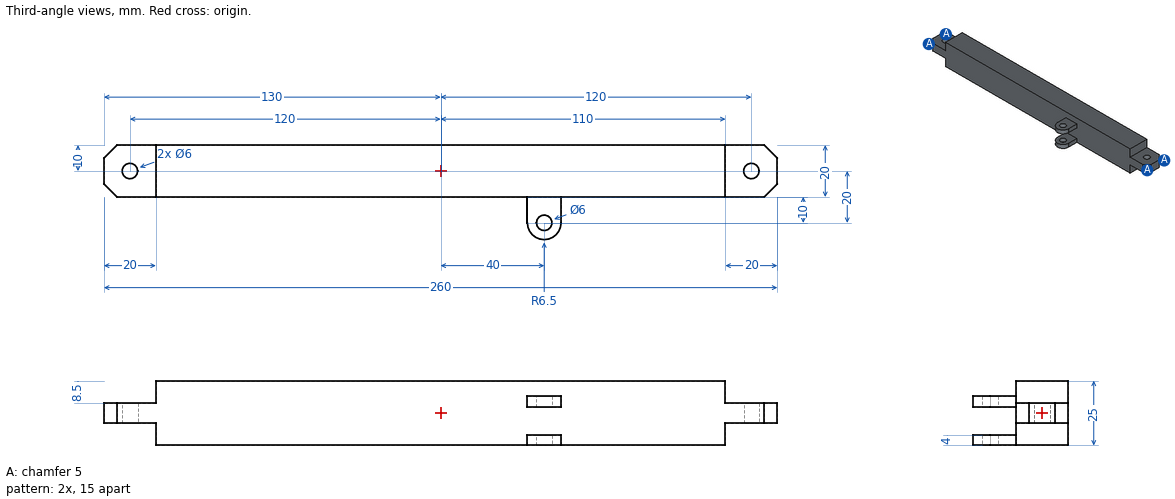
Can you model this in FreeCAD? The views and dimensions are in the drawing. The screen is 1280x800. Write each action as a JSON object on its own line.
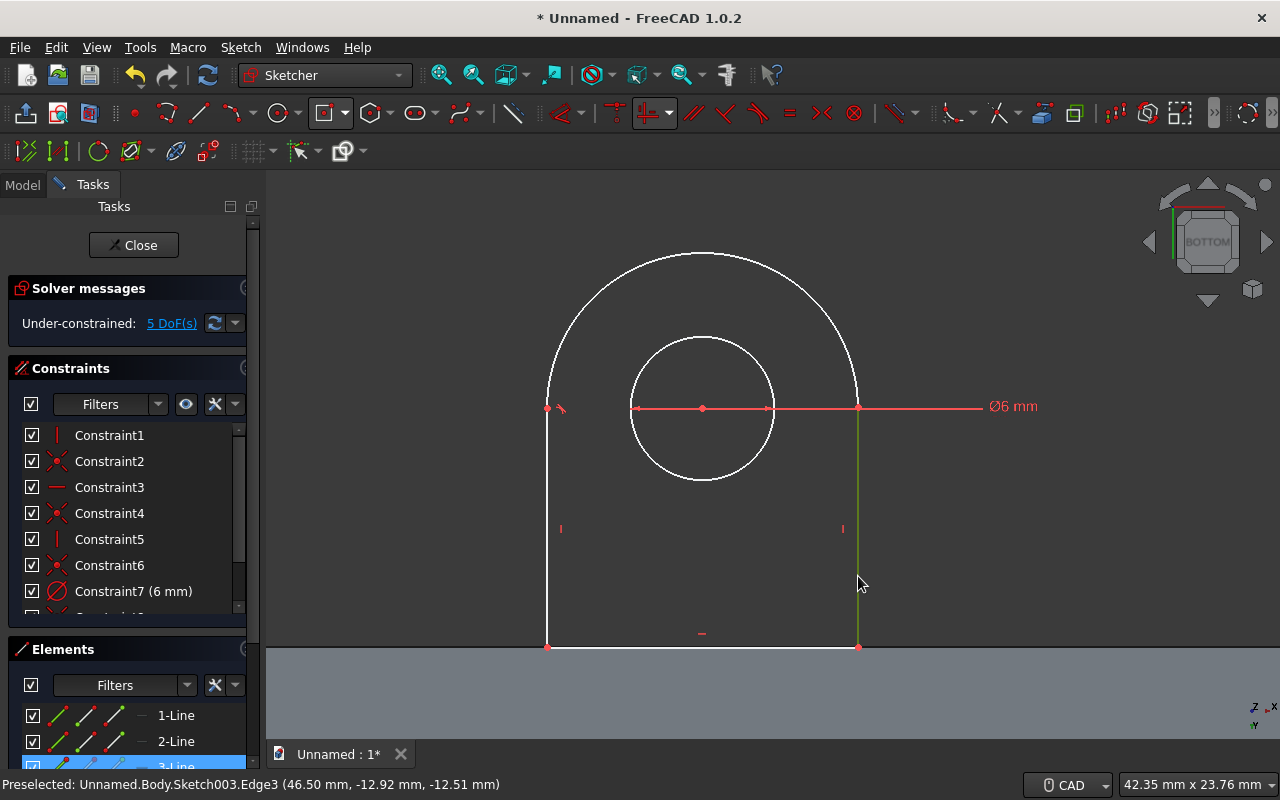
{"action": "left_click", "coordinate": [794, 282]}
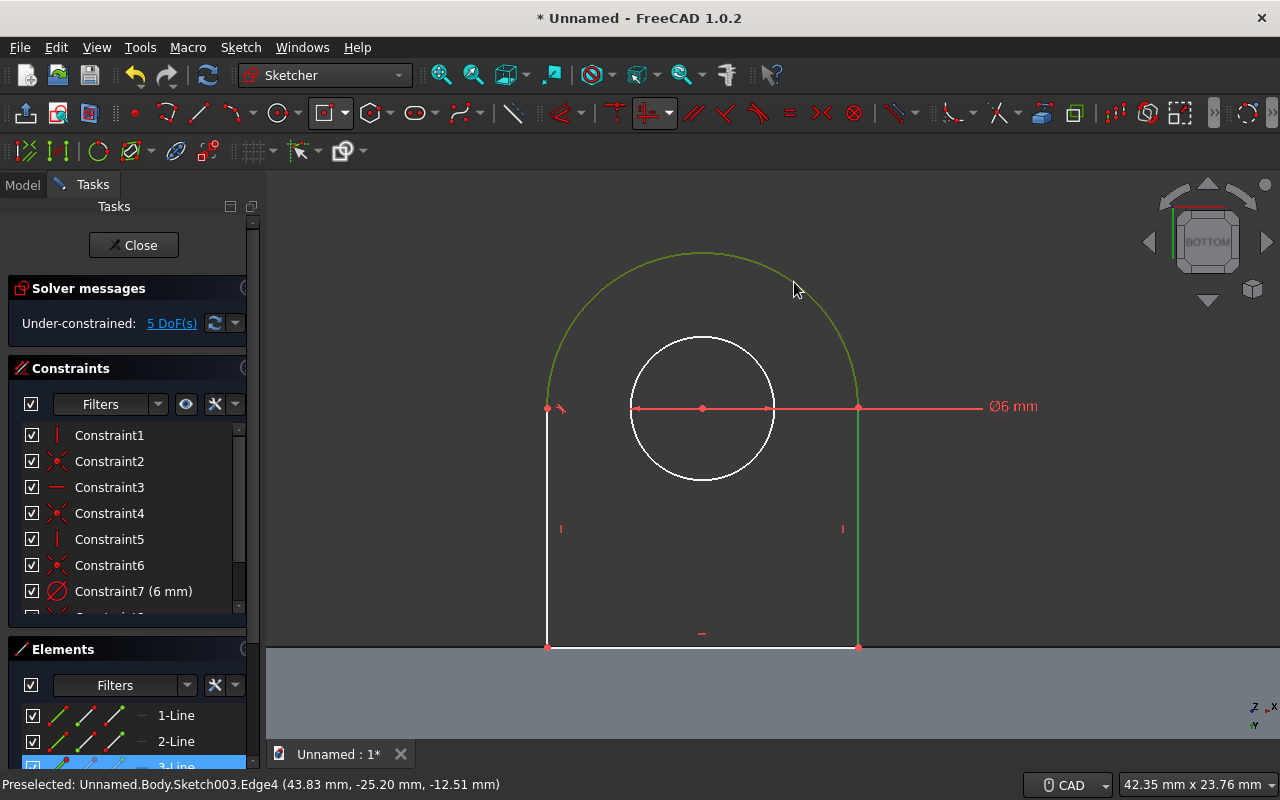
{"action": "left_click", "coordinate": [758, 114]}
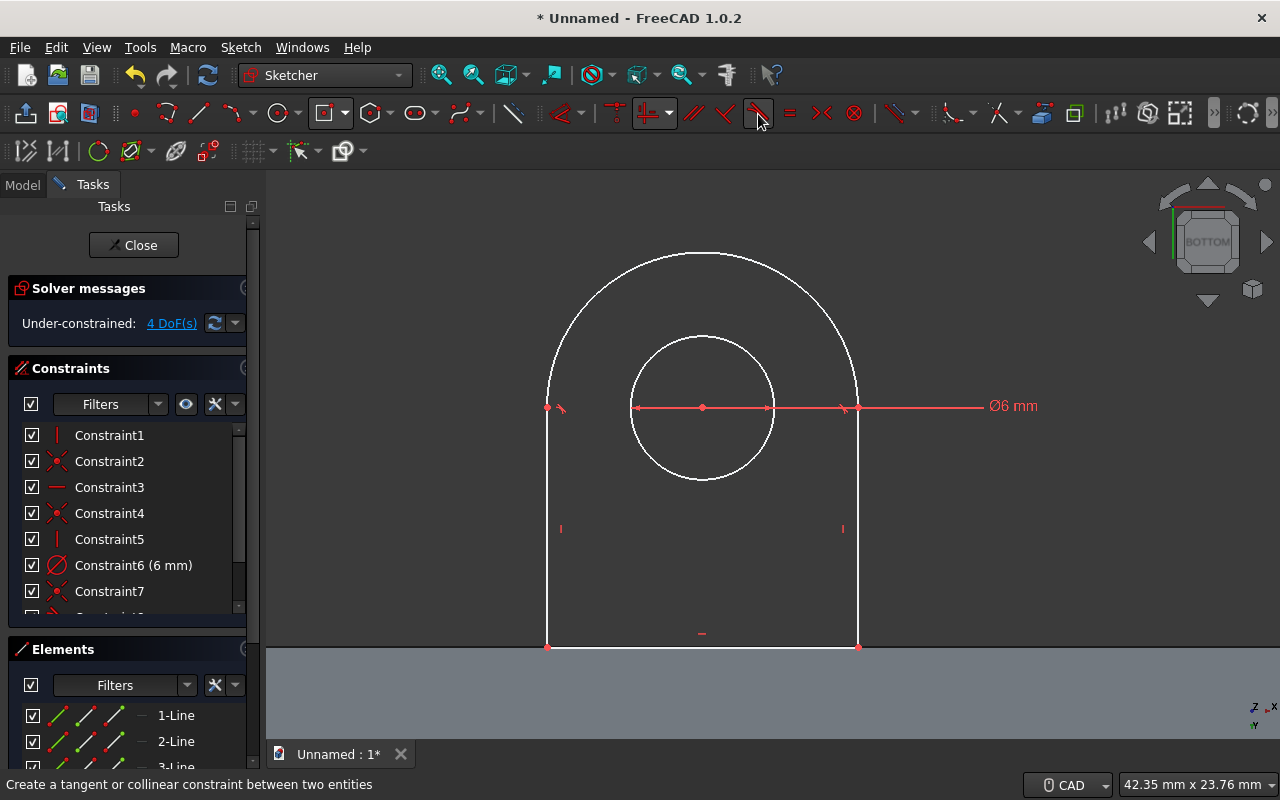
{"action": "left_click", "coordinate": [560, 114]}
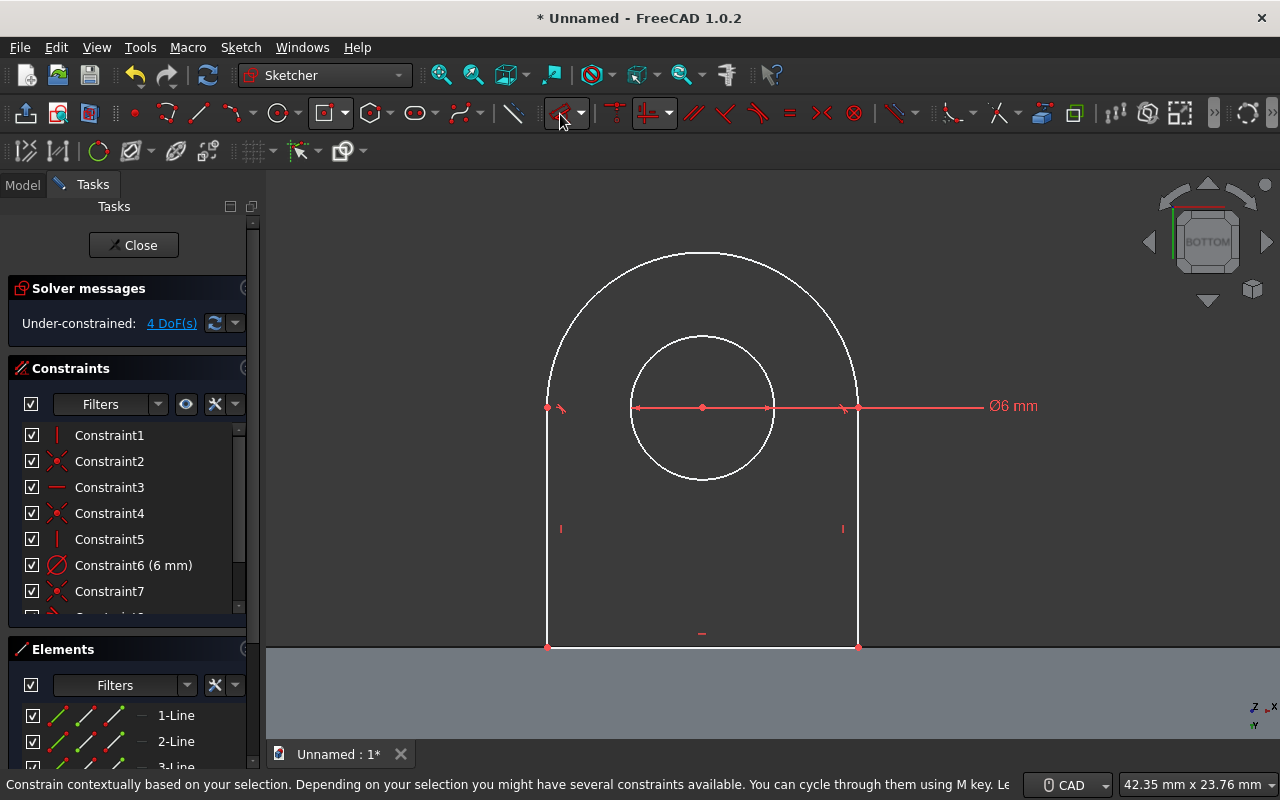
{"action": "left_click", "coordinate": [794, 282]}
{"action": "left_click", "coordinate": [813, 256]}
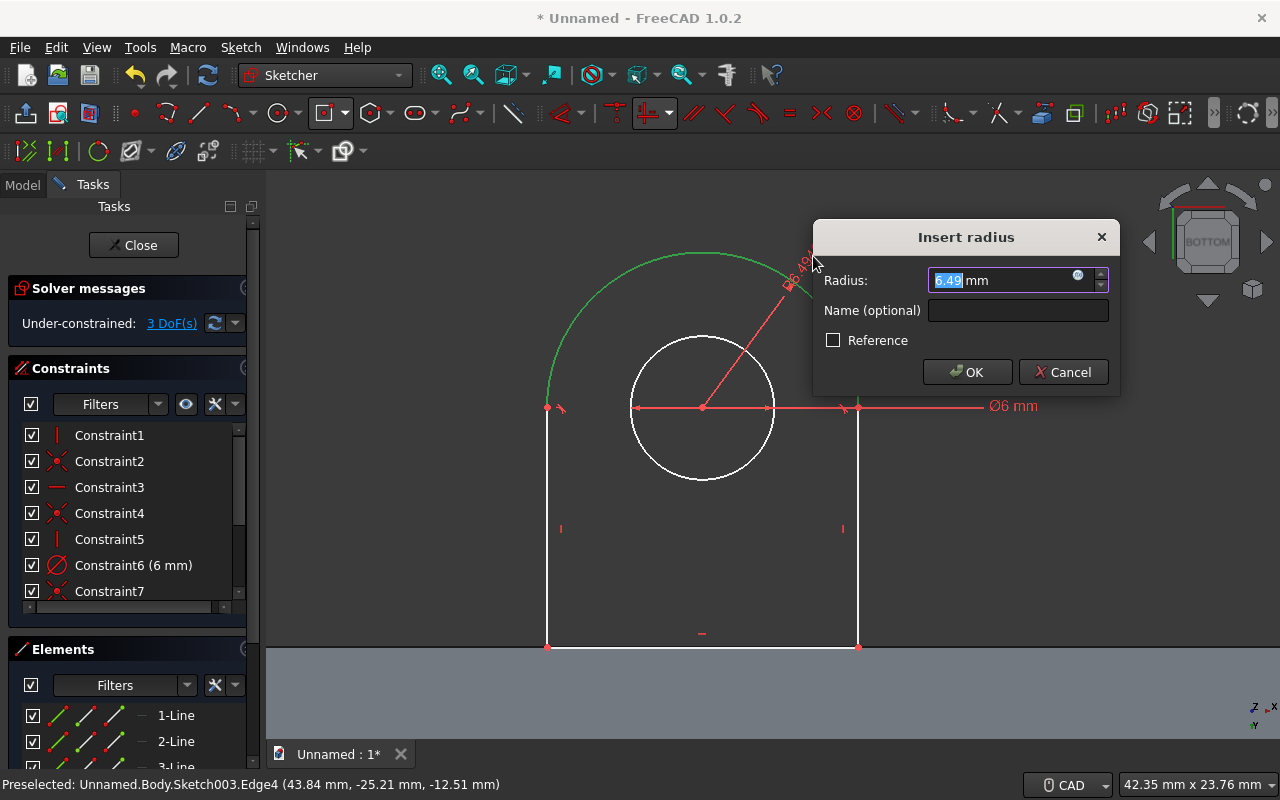
{"action": "type", "text": "6.5"}
{"action": "key", "text": "Return"}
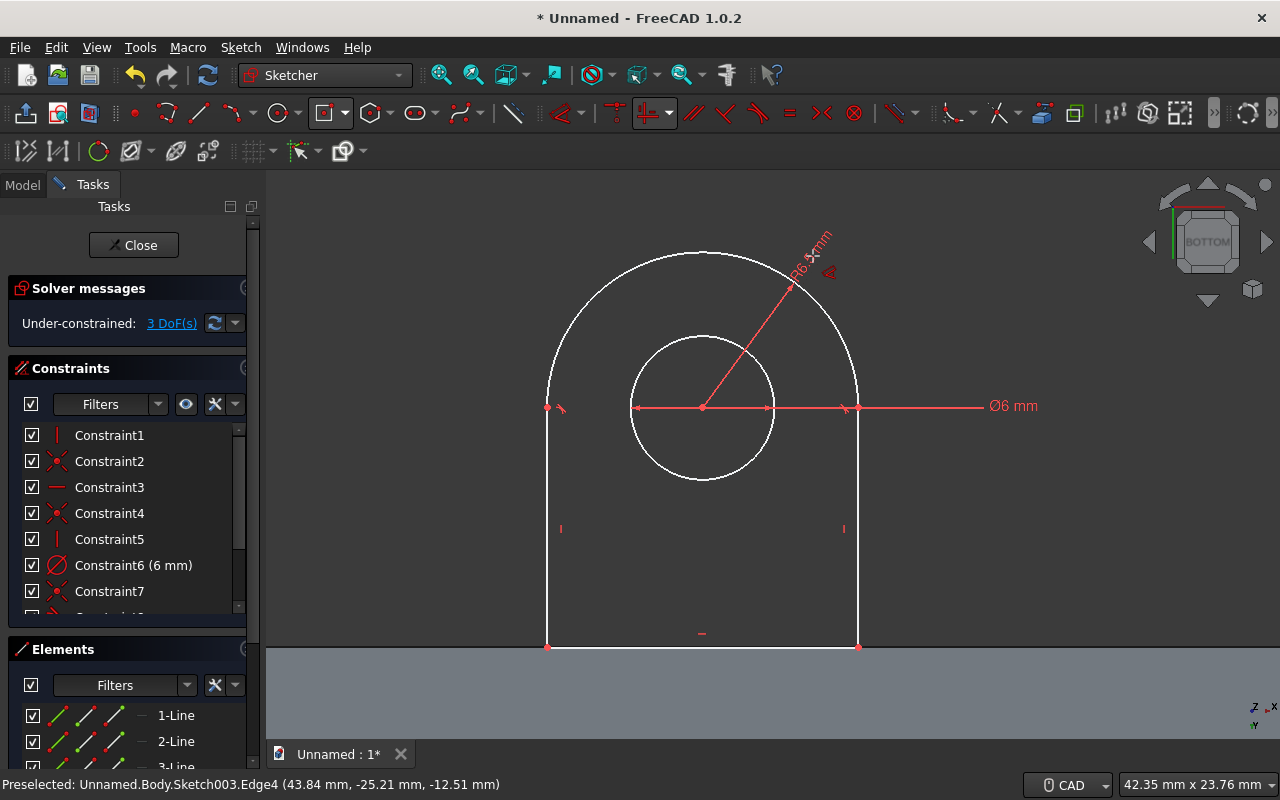
{"action": "left_click", "coordinate": [547, 480]}
{"action": "left_click", "coordinate": [513, 528]}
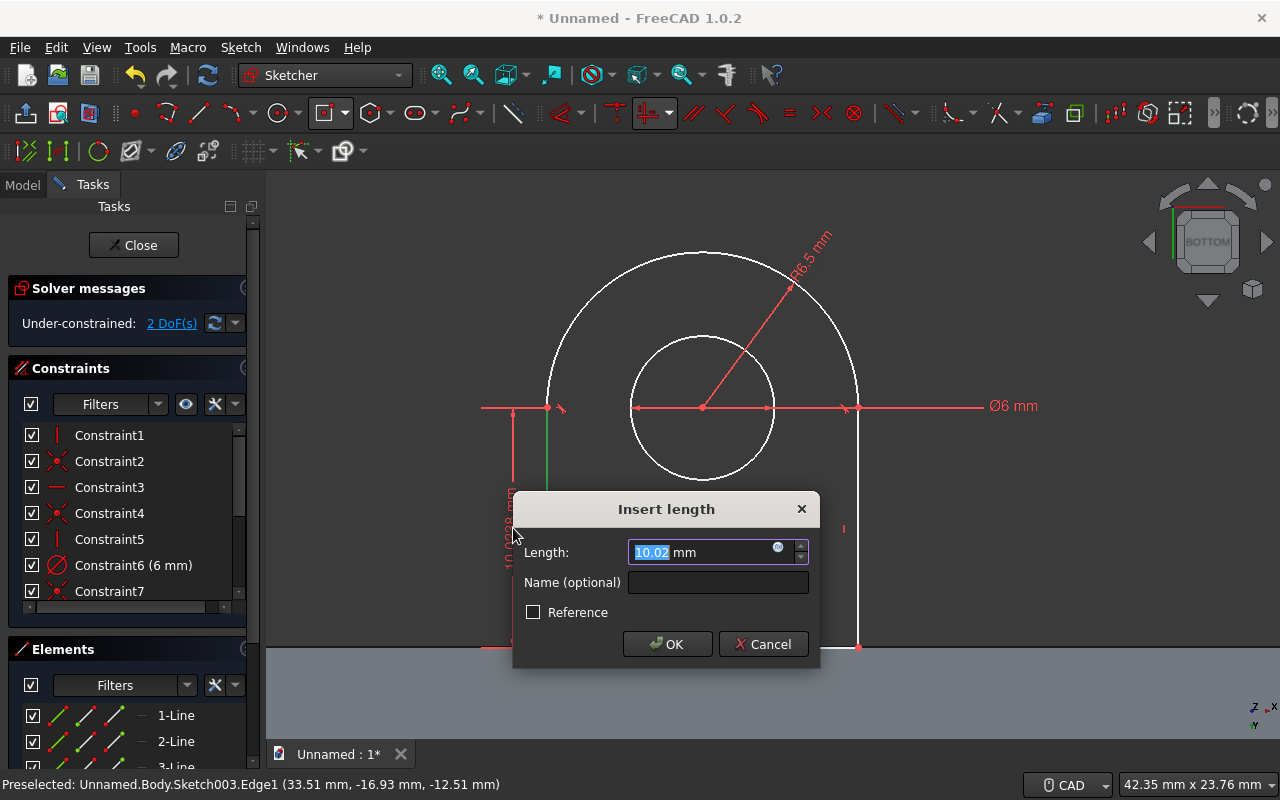
{"action": "type", "text": "10"}
{"action": "key", "text": "Return"}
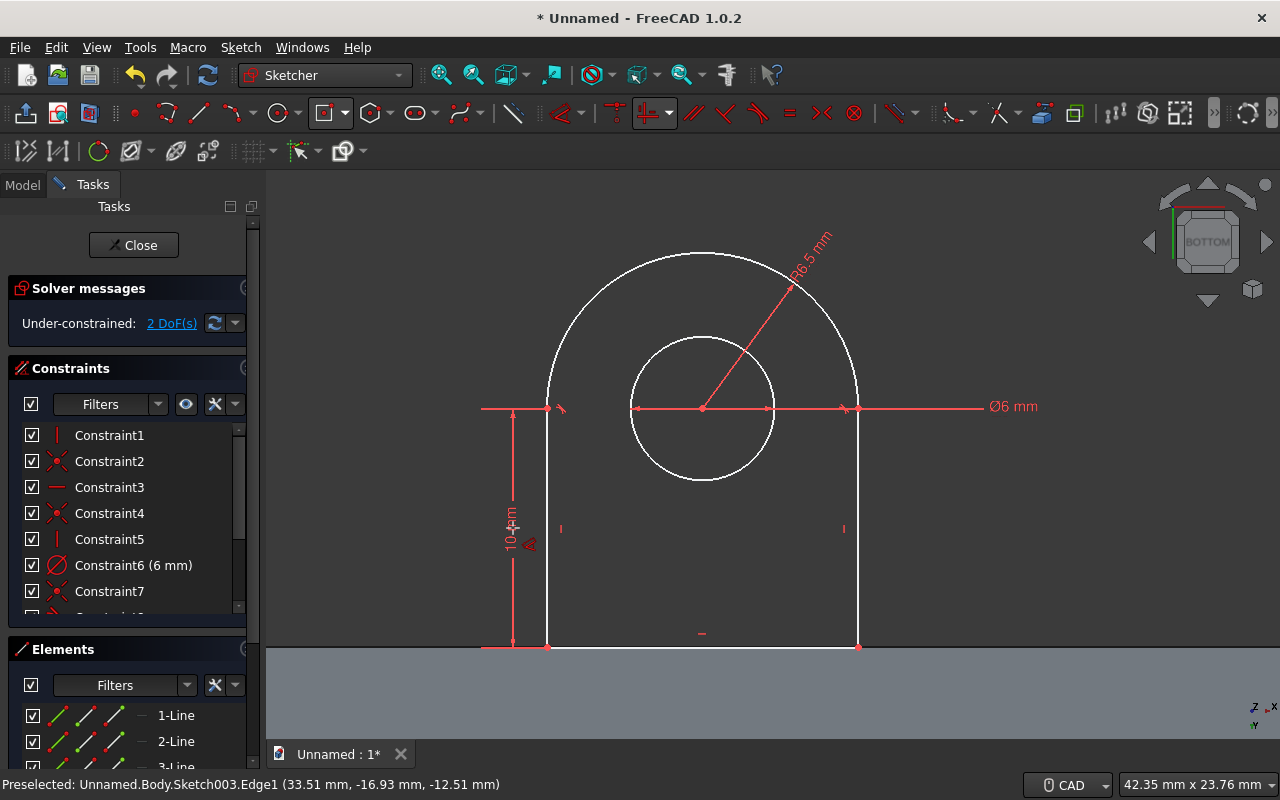
{"action": "left_click", "coordinate": [703, 409]}
{"action": "left_click", "coordinate": [498, 375]}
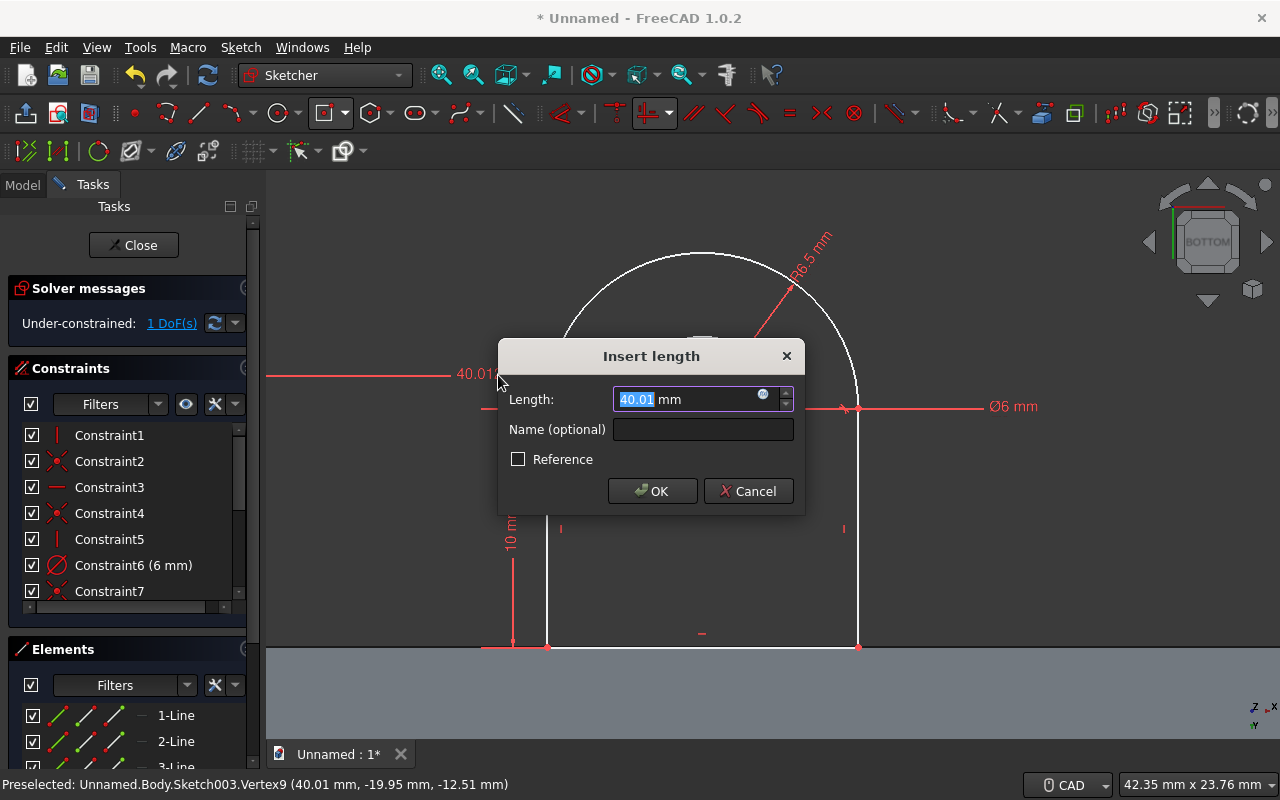
{"action": "type", "text": "40"}
{"action": "key", "text": "Return"}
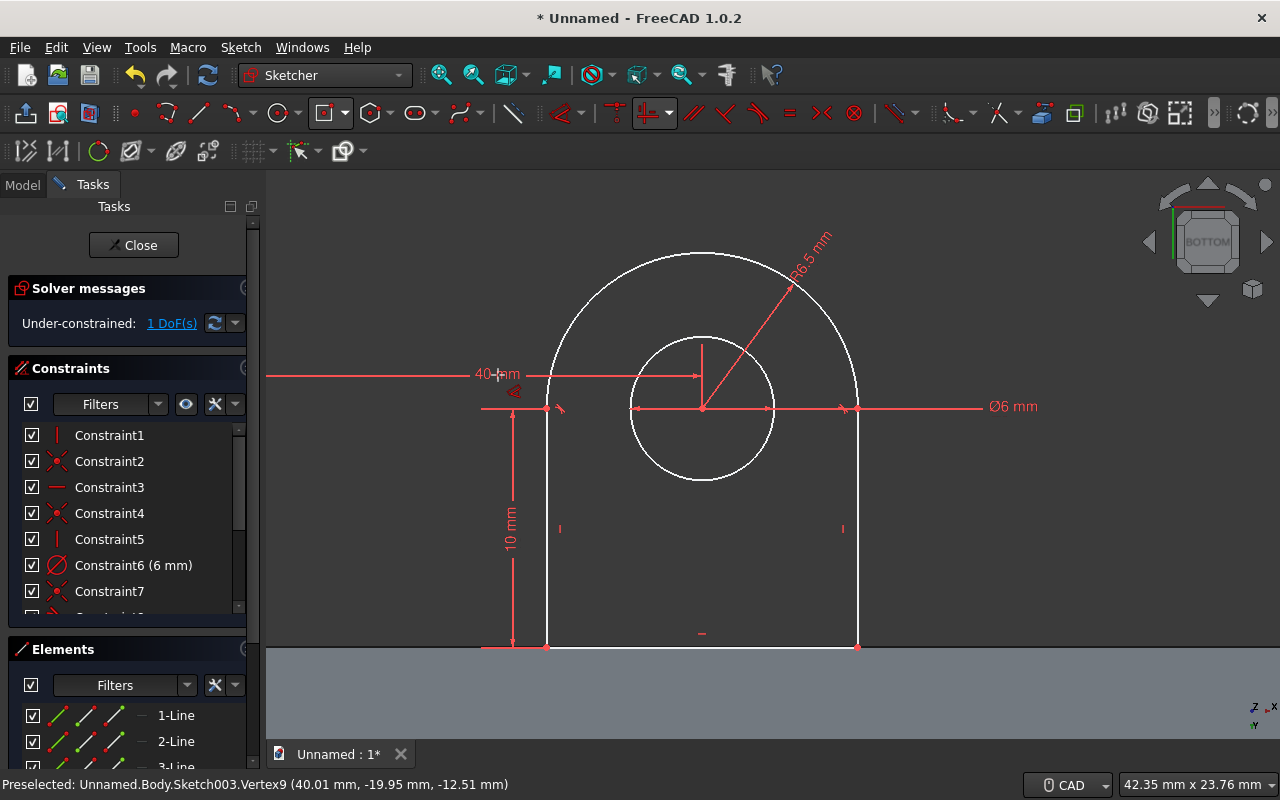
{"action": "left_click", "coordinate": [702, 409]}
{"action": "left_click", "coordinate": [736, 560]}